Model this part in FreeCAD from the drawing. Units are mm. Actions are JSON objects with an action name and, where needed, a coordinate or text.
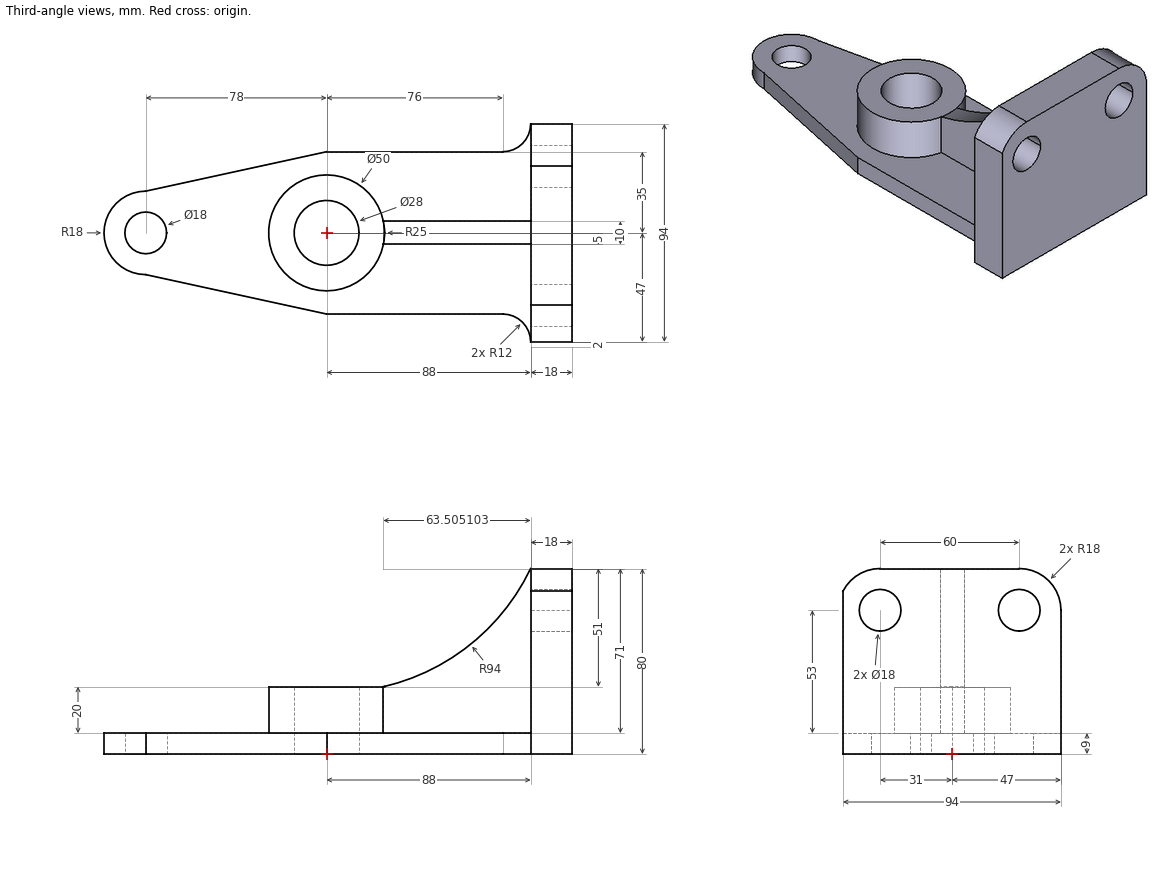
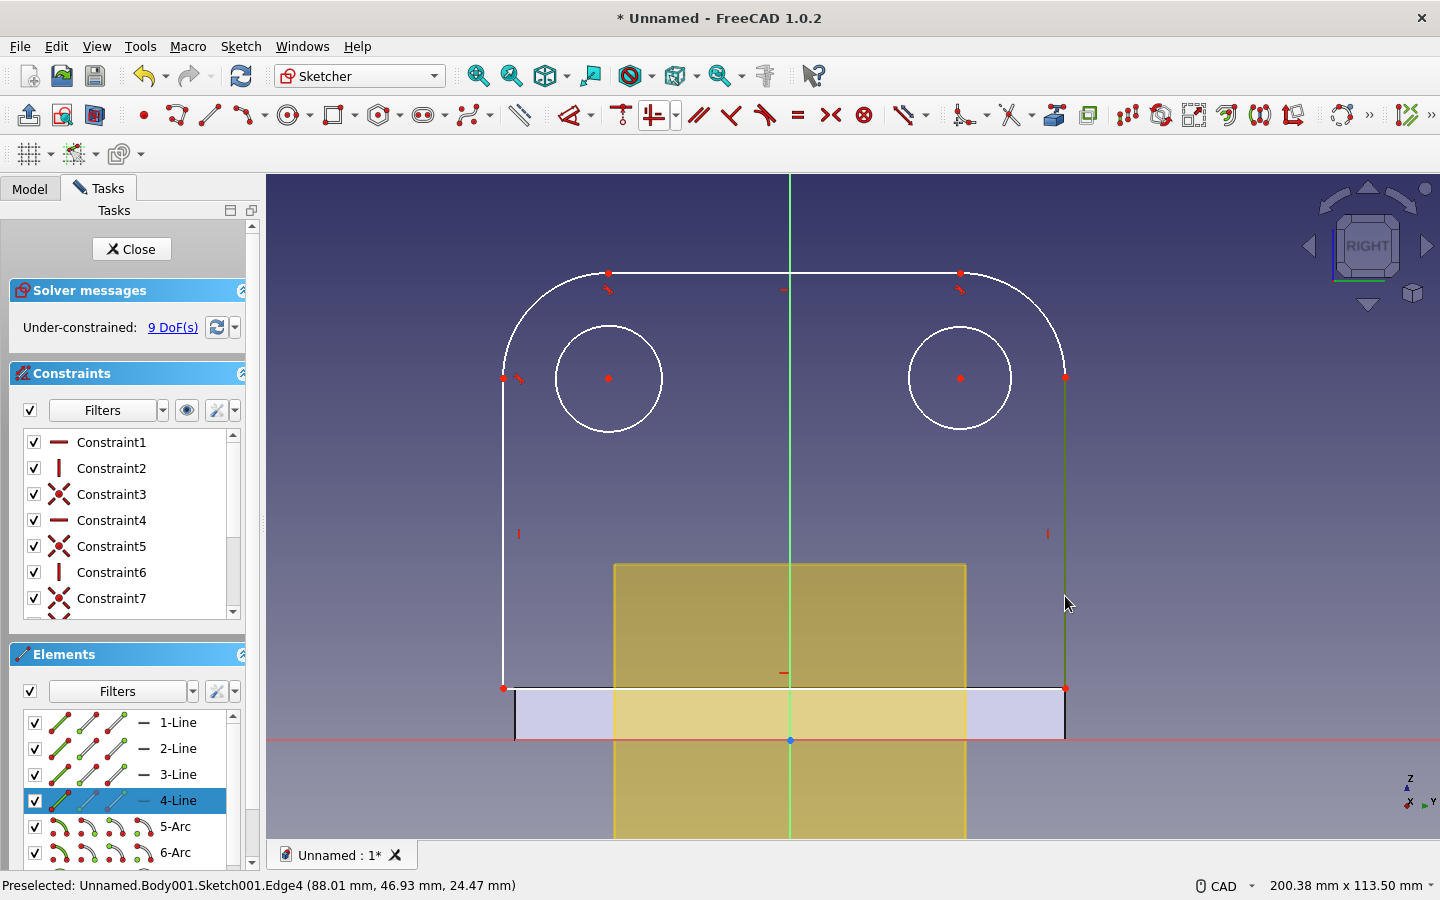
{"action": "left_click", "coordinate": [1054, 330]}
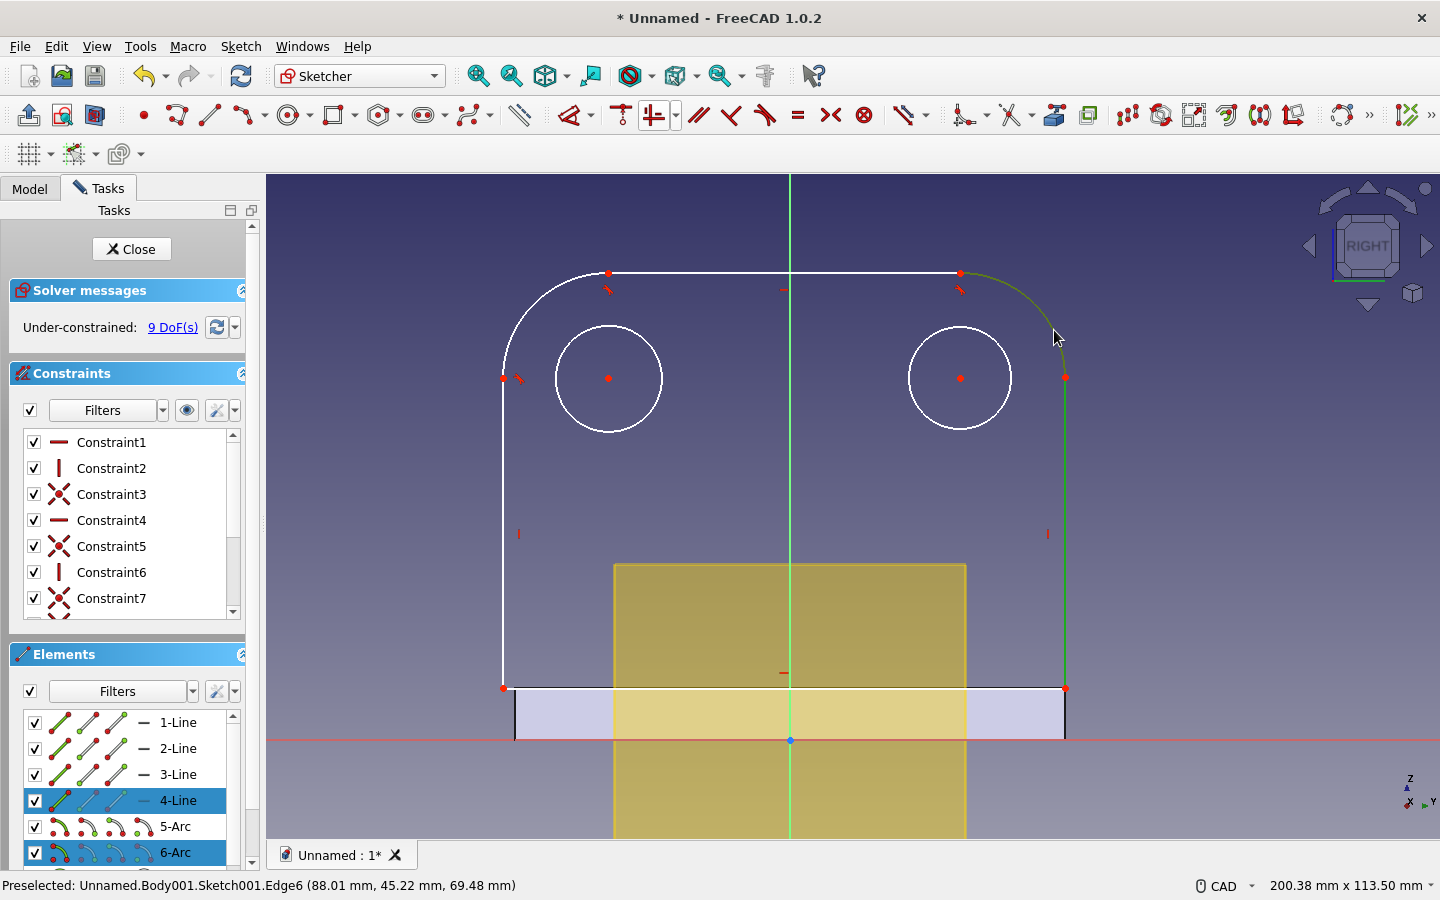
{"action": "left_click", "coordinate": [765, 116]}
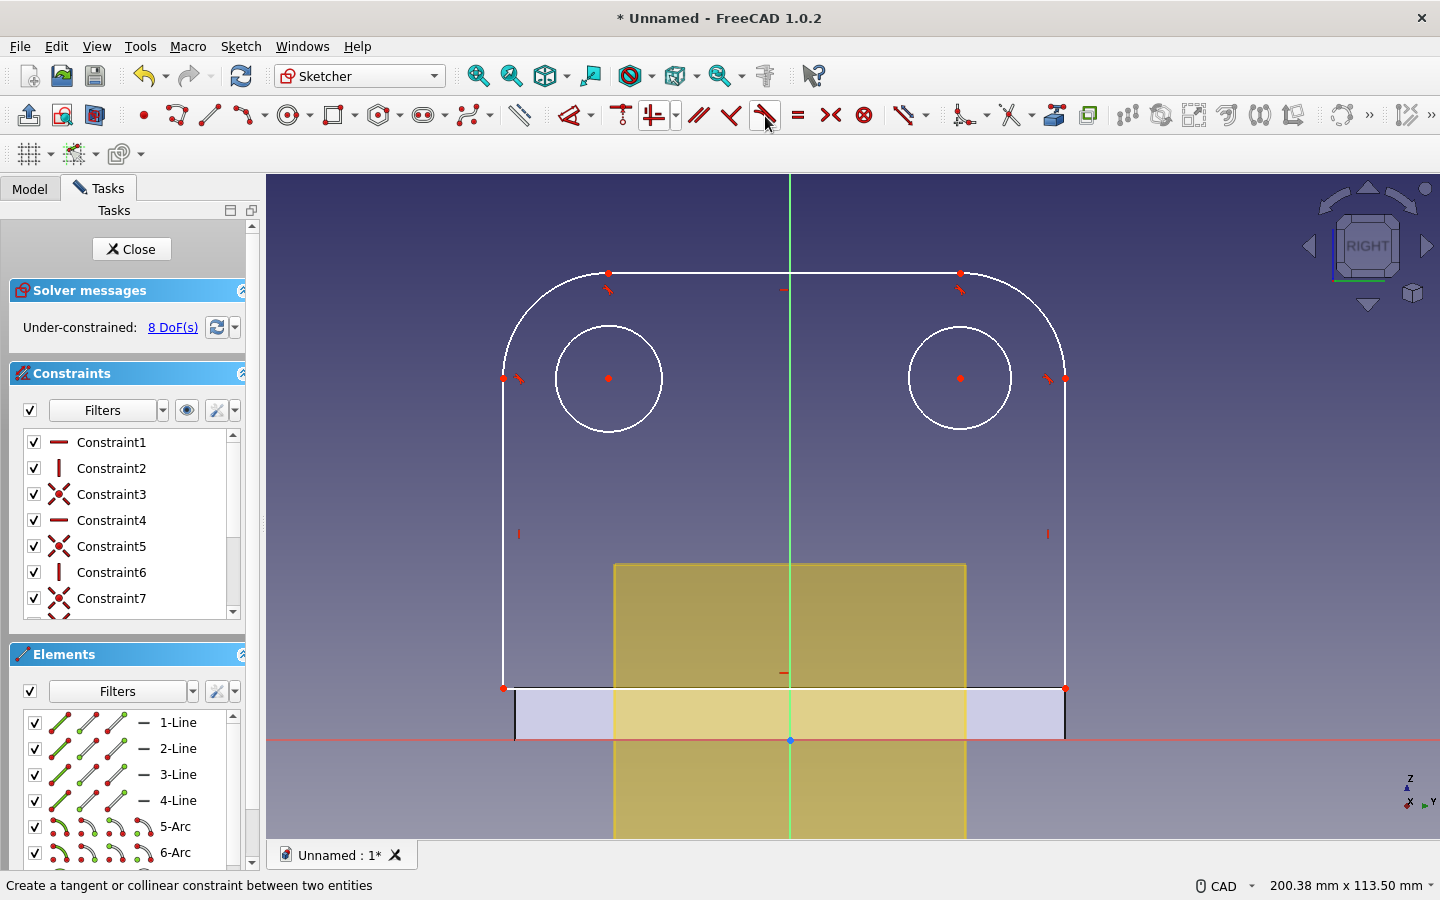
{"action": "left_click", "coordinate": [561, 285]}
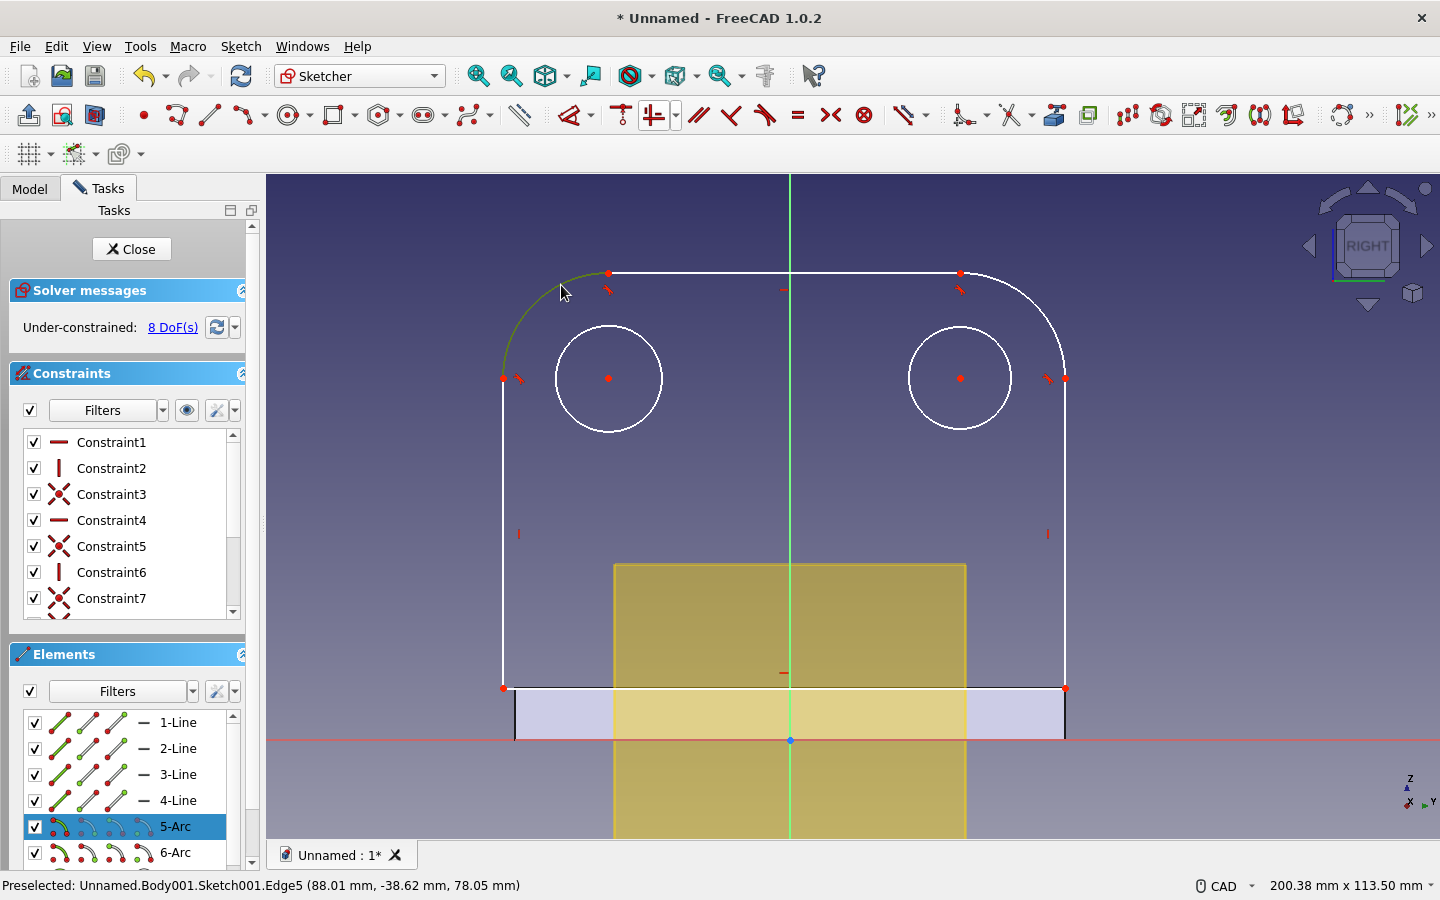
{"action": "left_click", "coordinate": [1054, 330]}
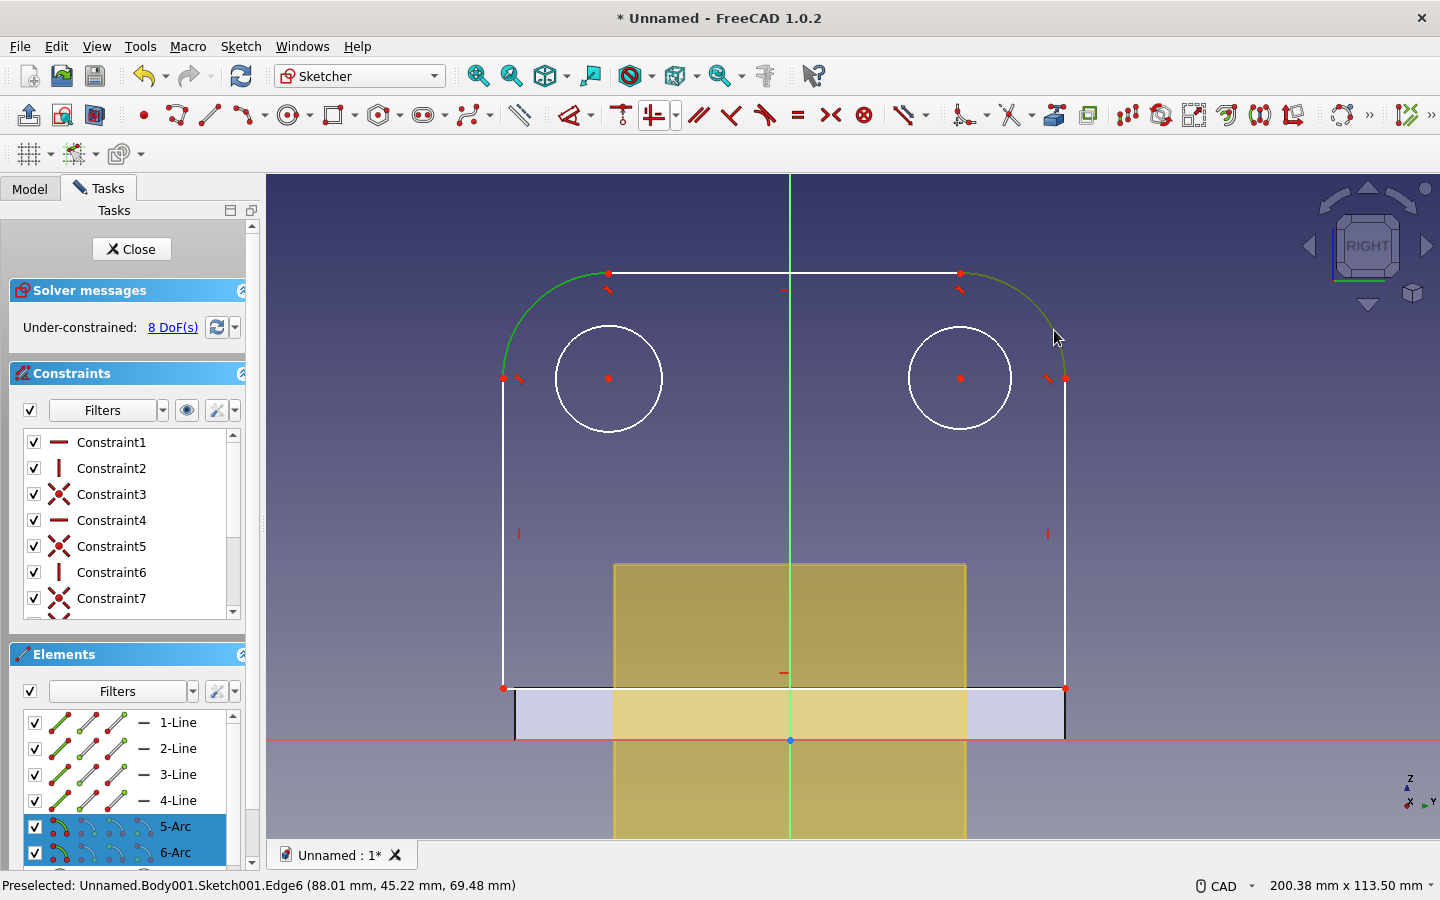
{"action": "key", "text": "e"}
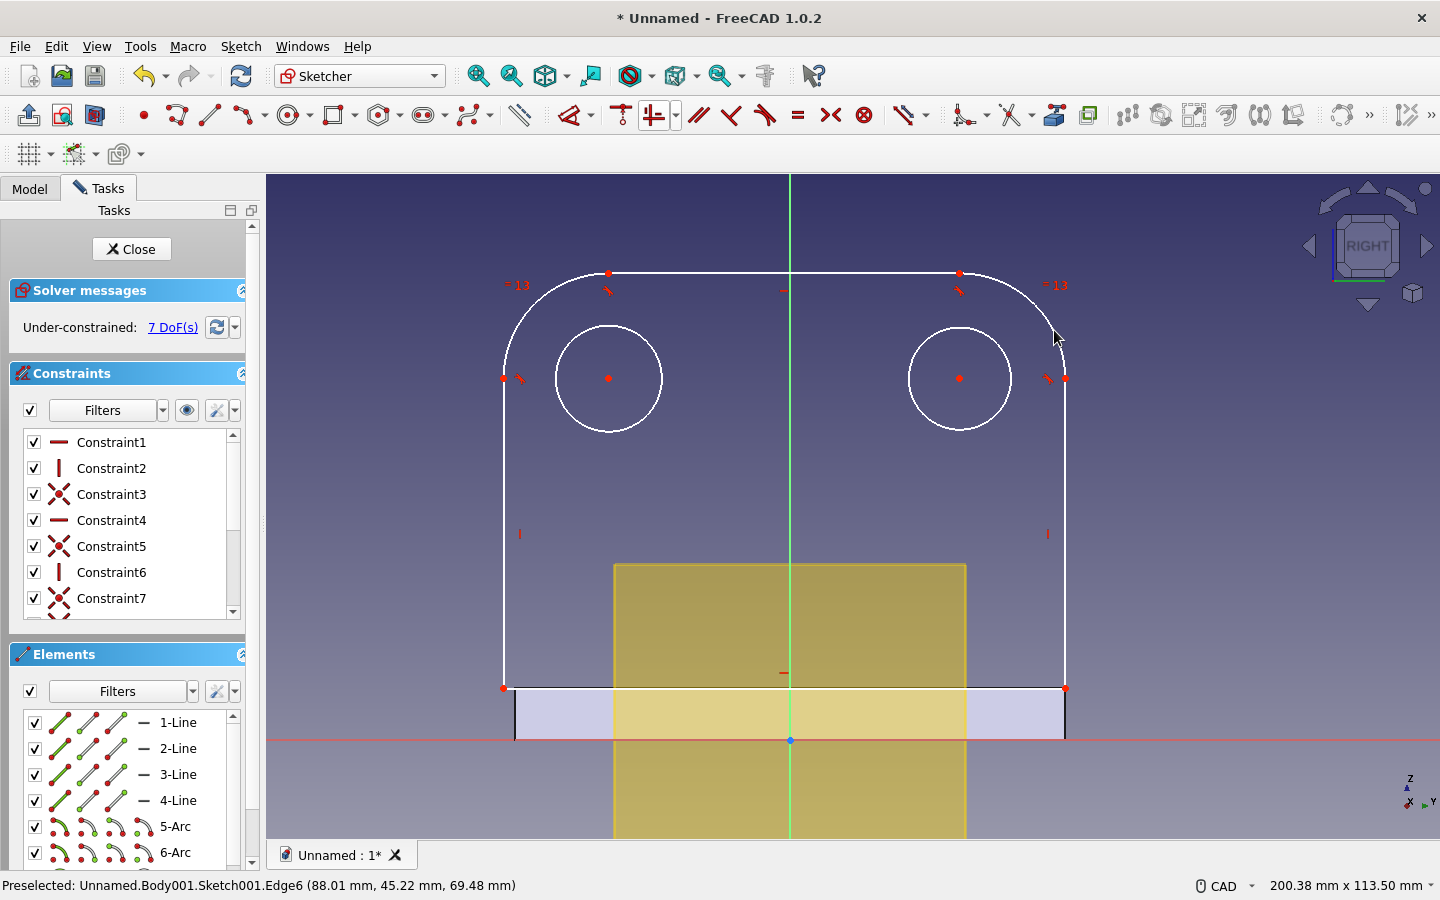
{"action": "left_click", "coordinate": [646, 341]}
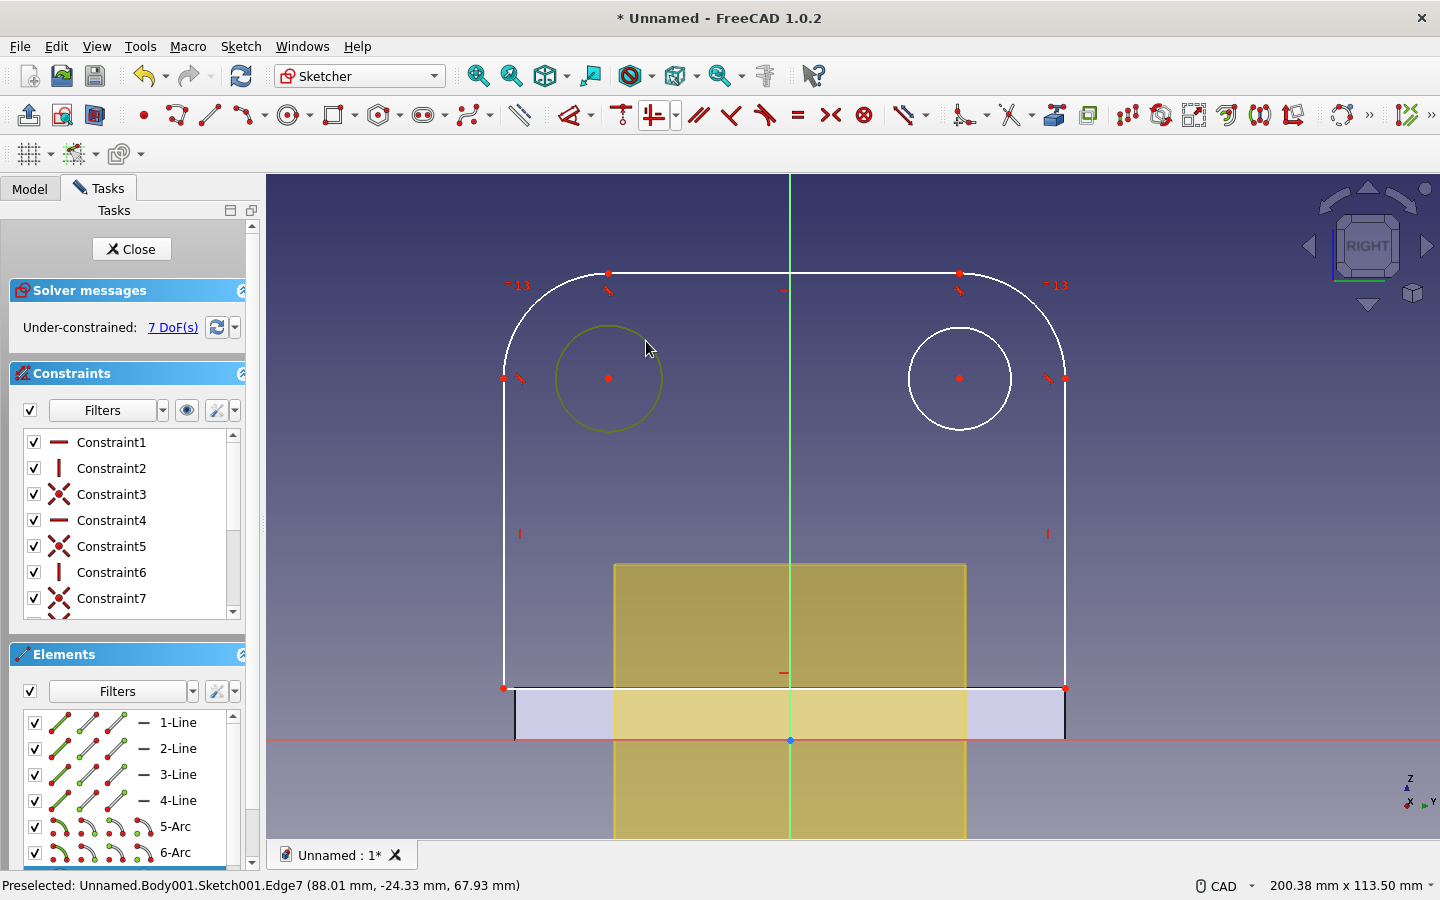
{"action": "left_click", "coordinate": [996, 342]}